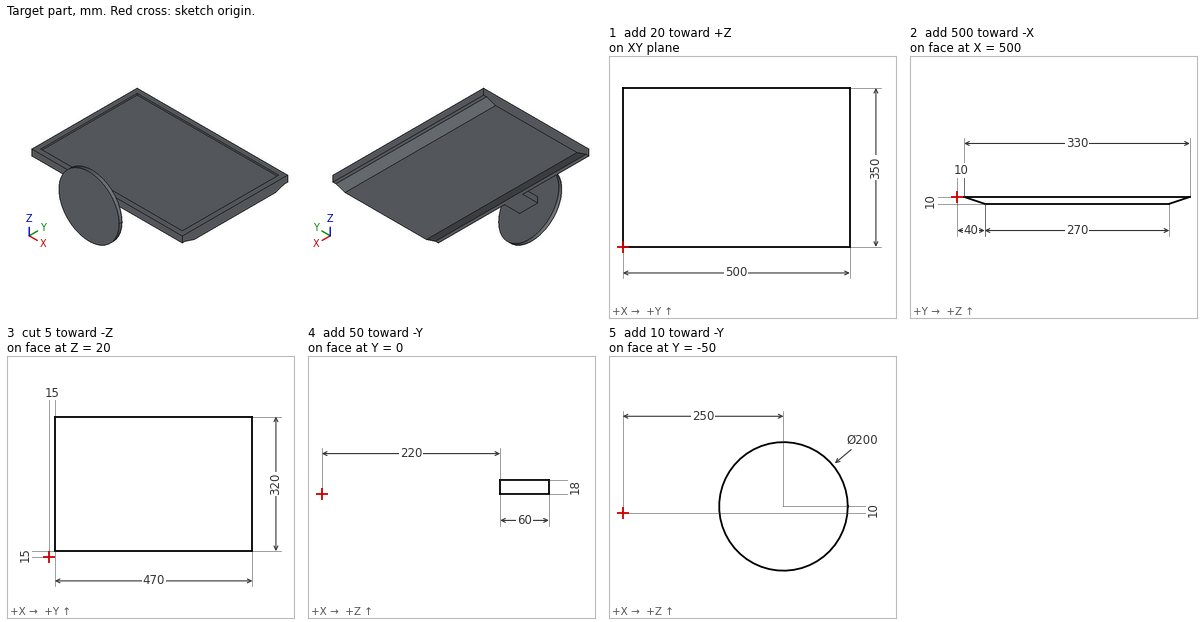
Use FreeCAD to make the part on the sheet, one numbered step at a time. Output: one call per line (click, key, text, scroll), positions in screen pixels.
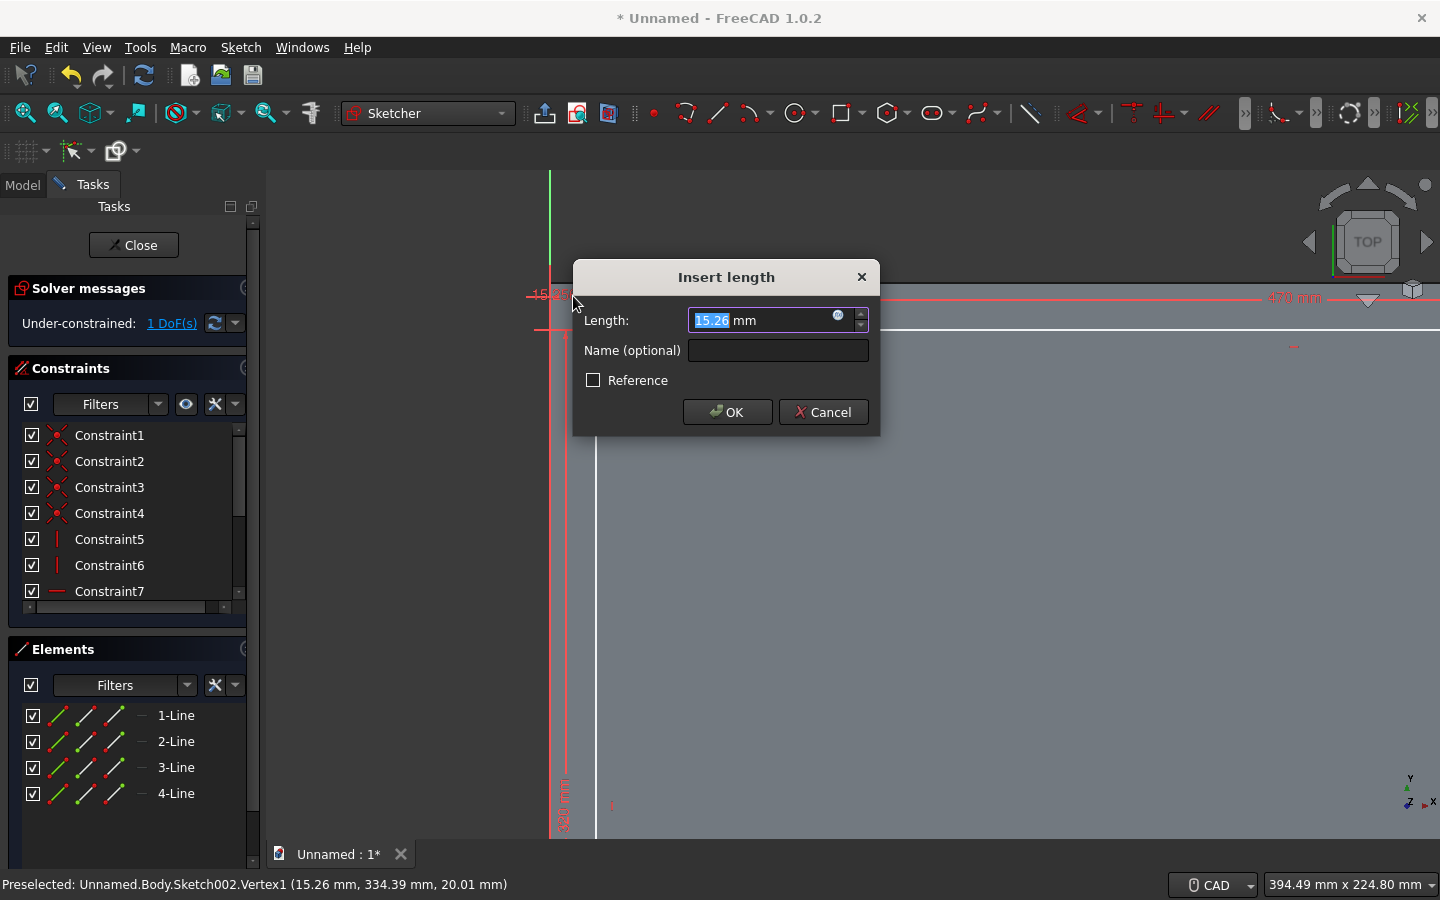
text(15)
key(Return)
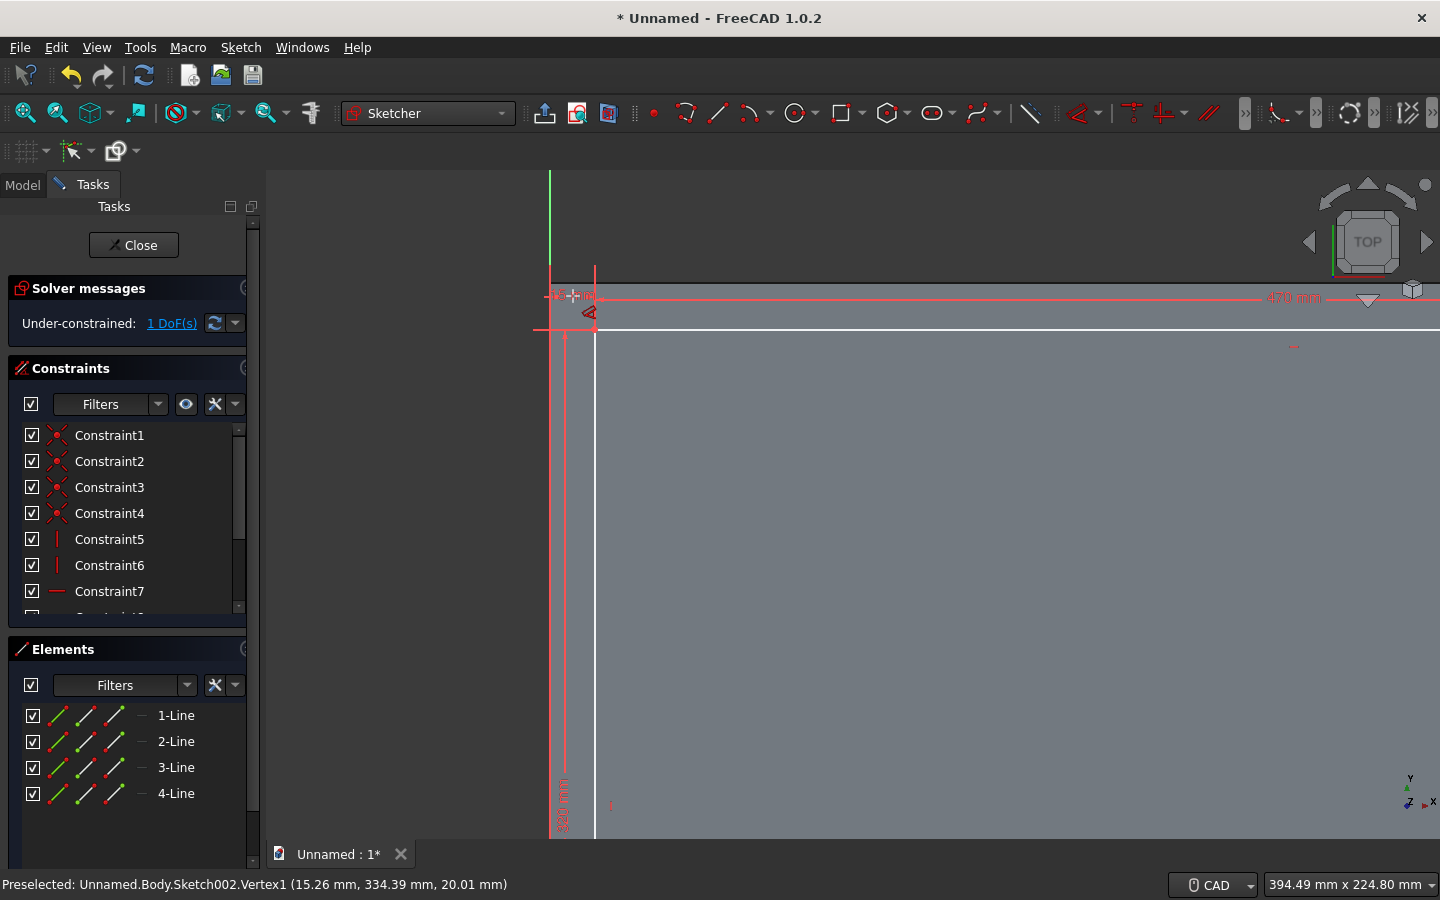
scroll(387, 242, down, 4)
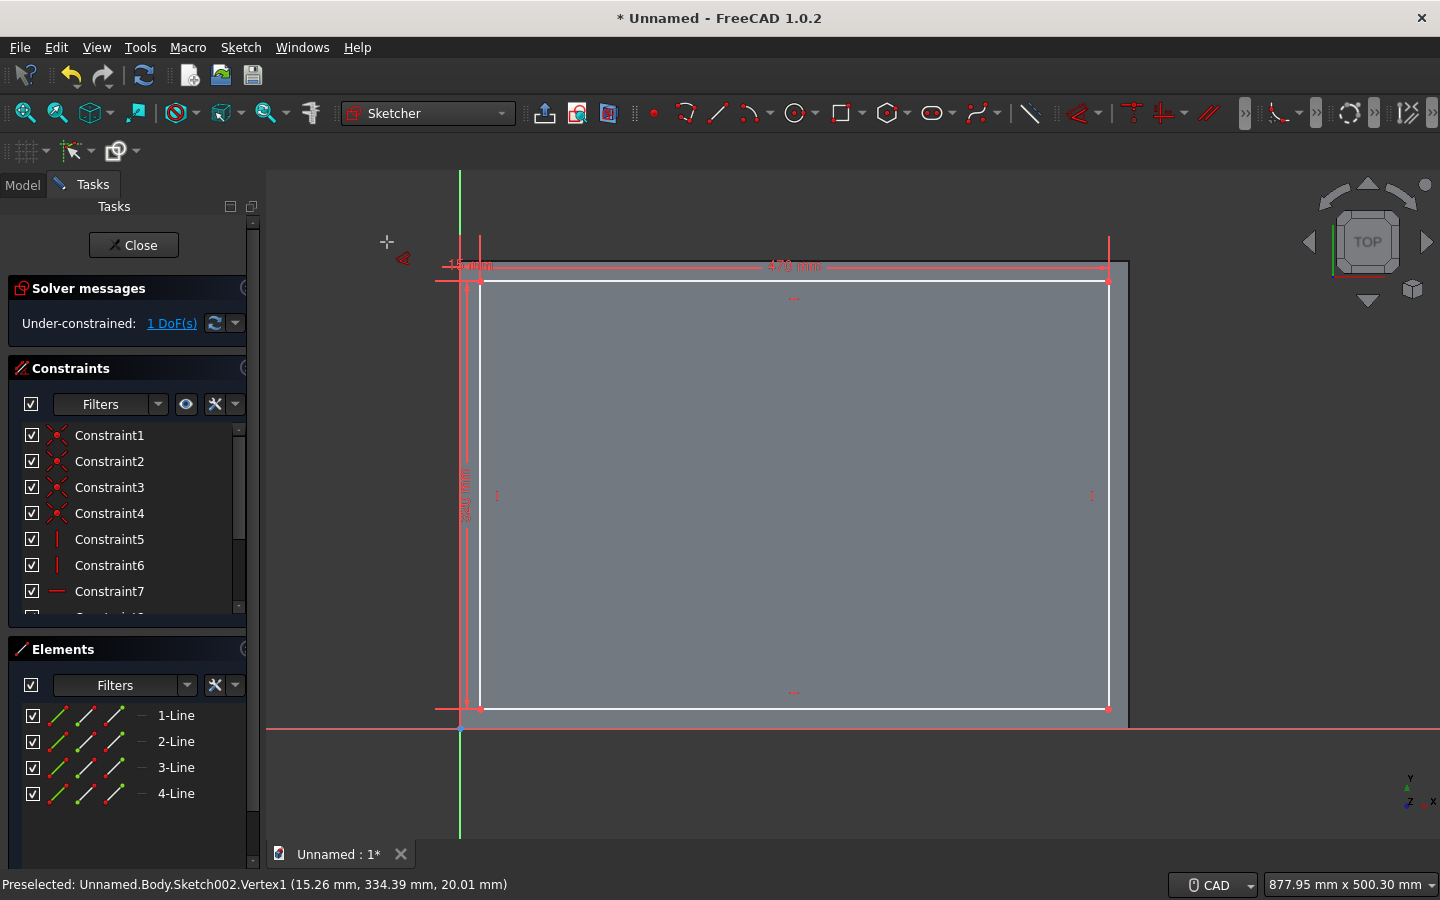
scroll(480, 709, up, 4)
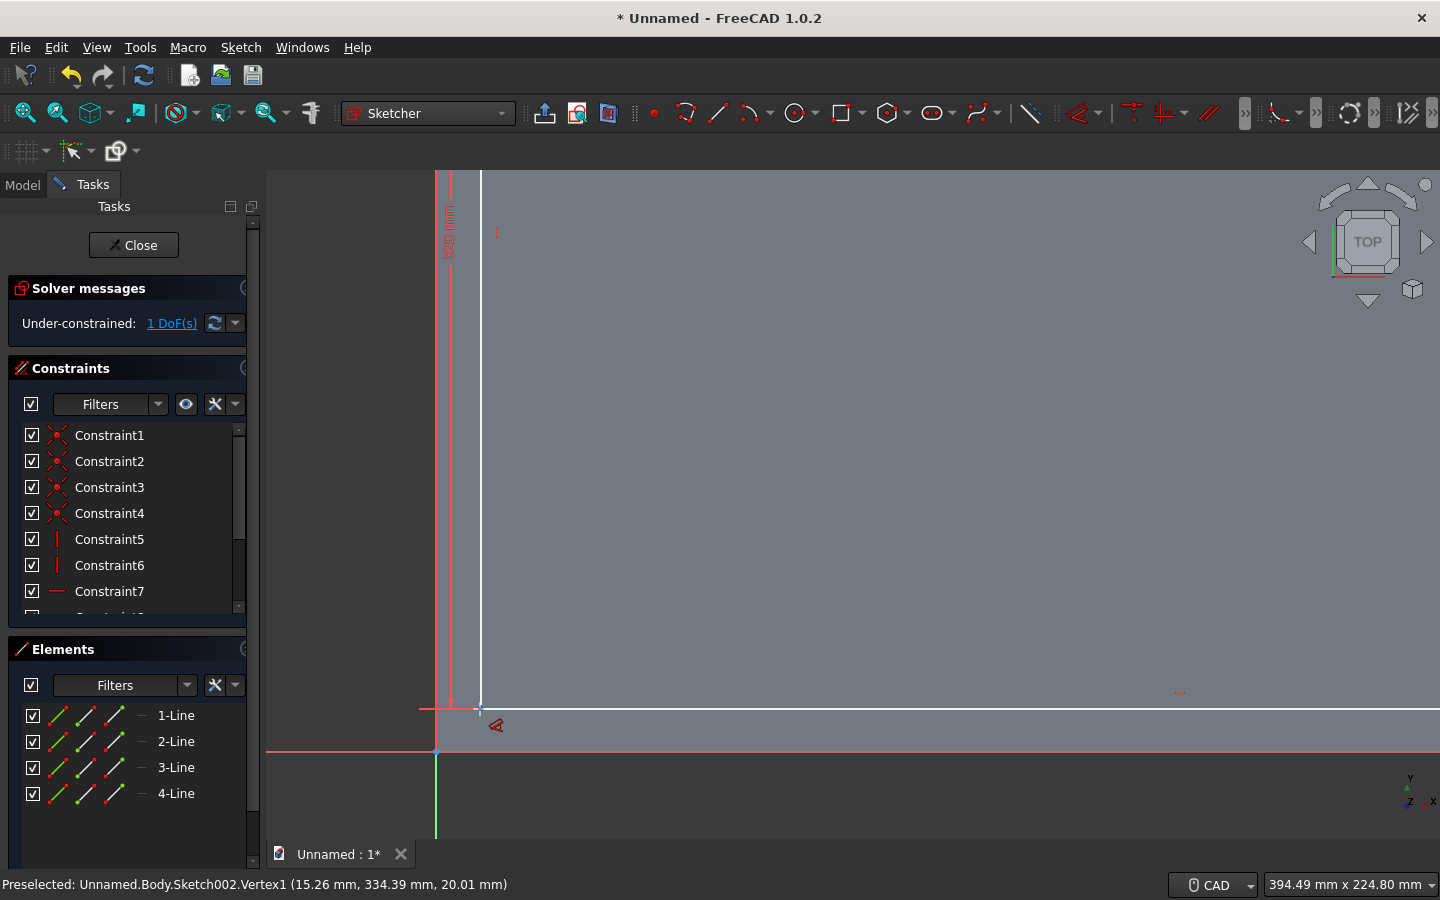
click(481, 709)
click(402, 730)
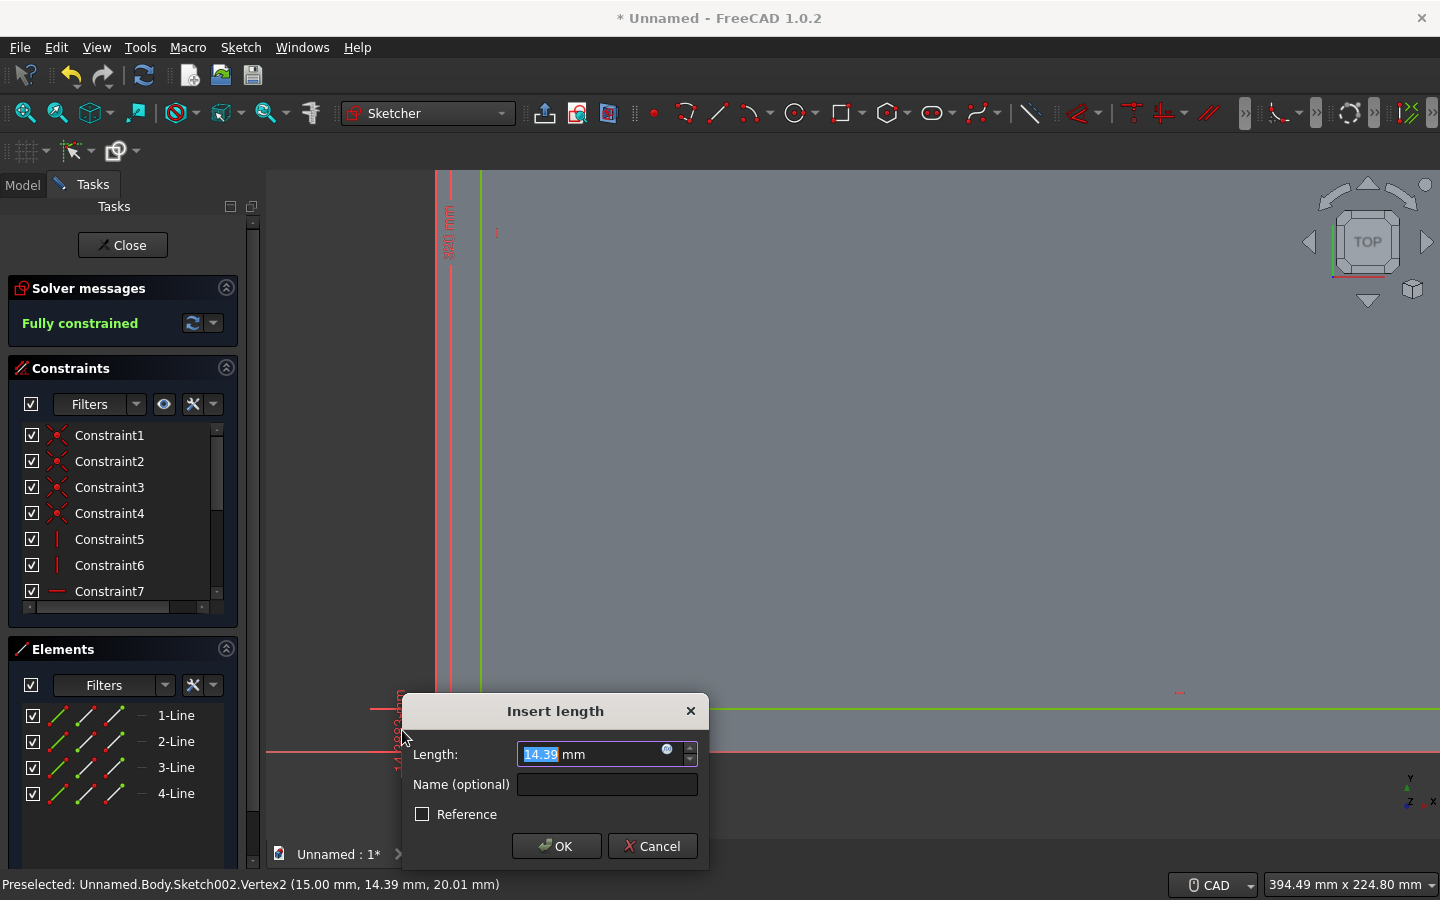
text(15)
key(Return)
key(Escape)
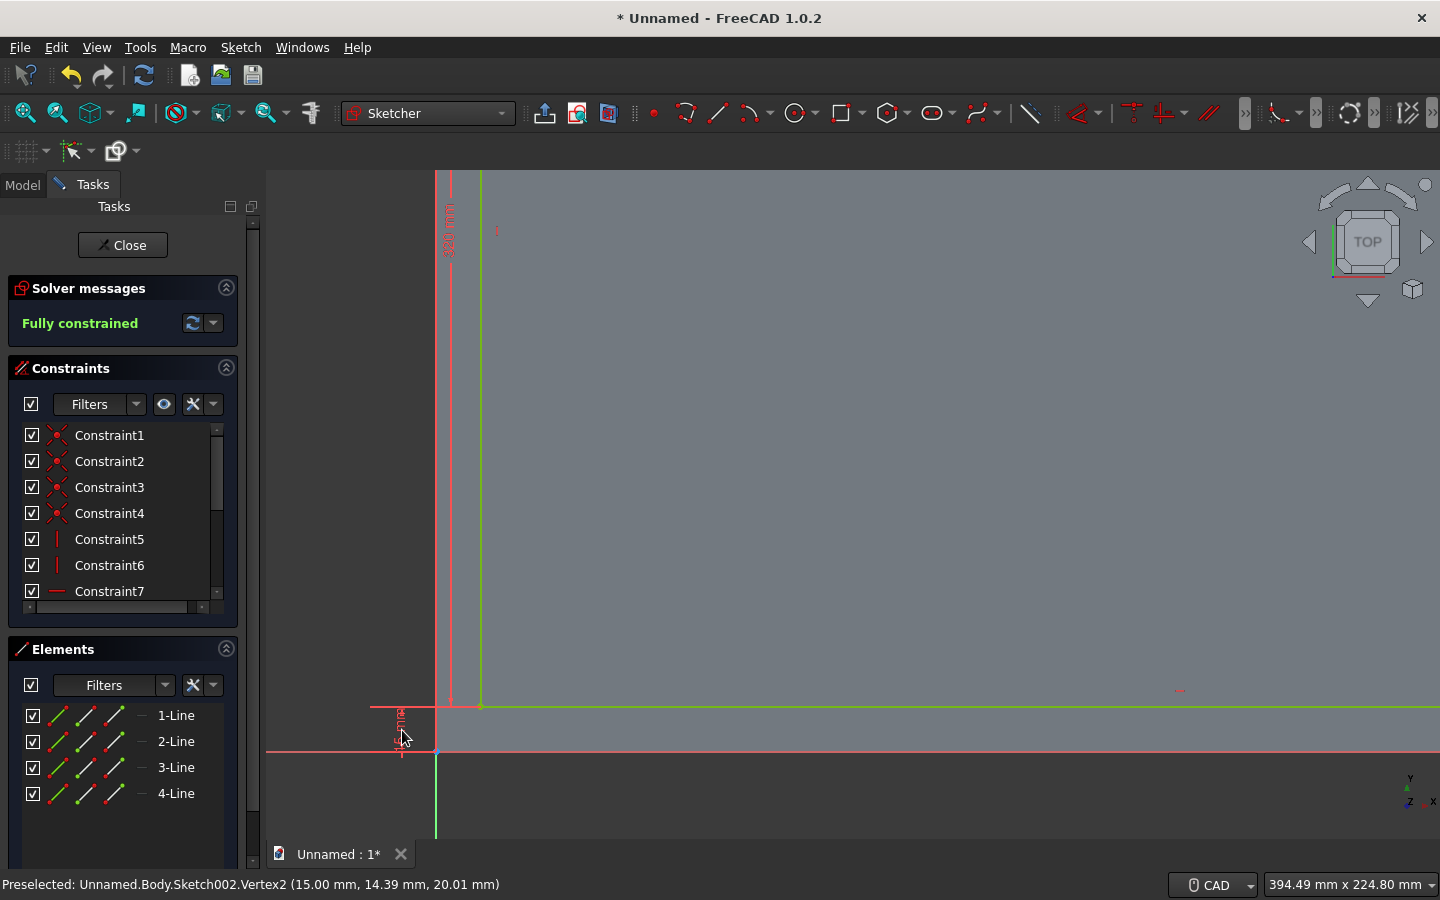
click(123, 245)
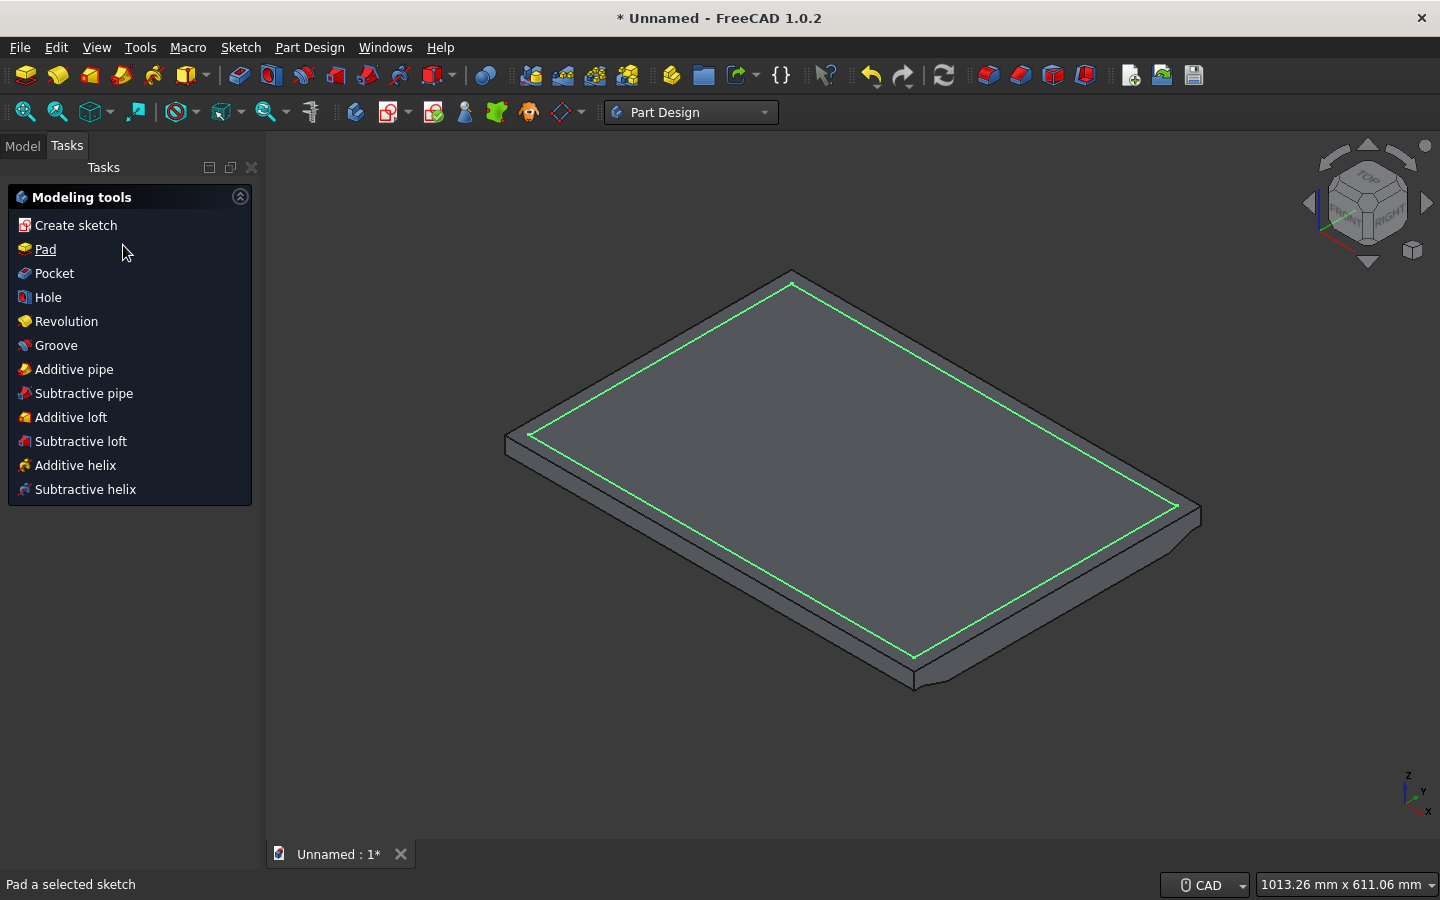
click(240, 76)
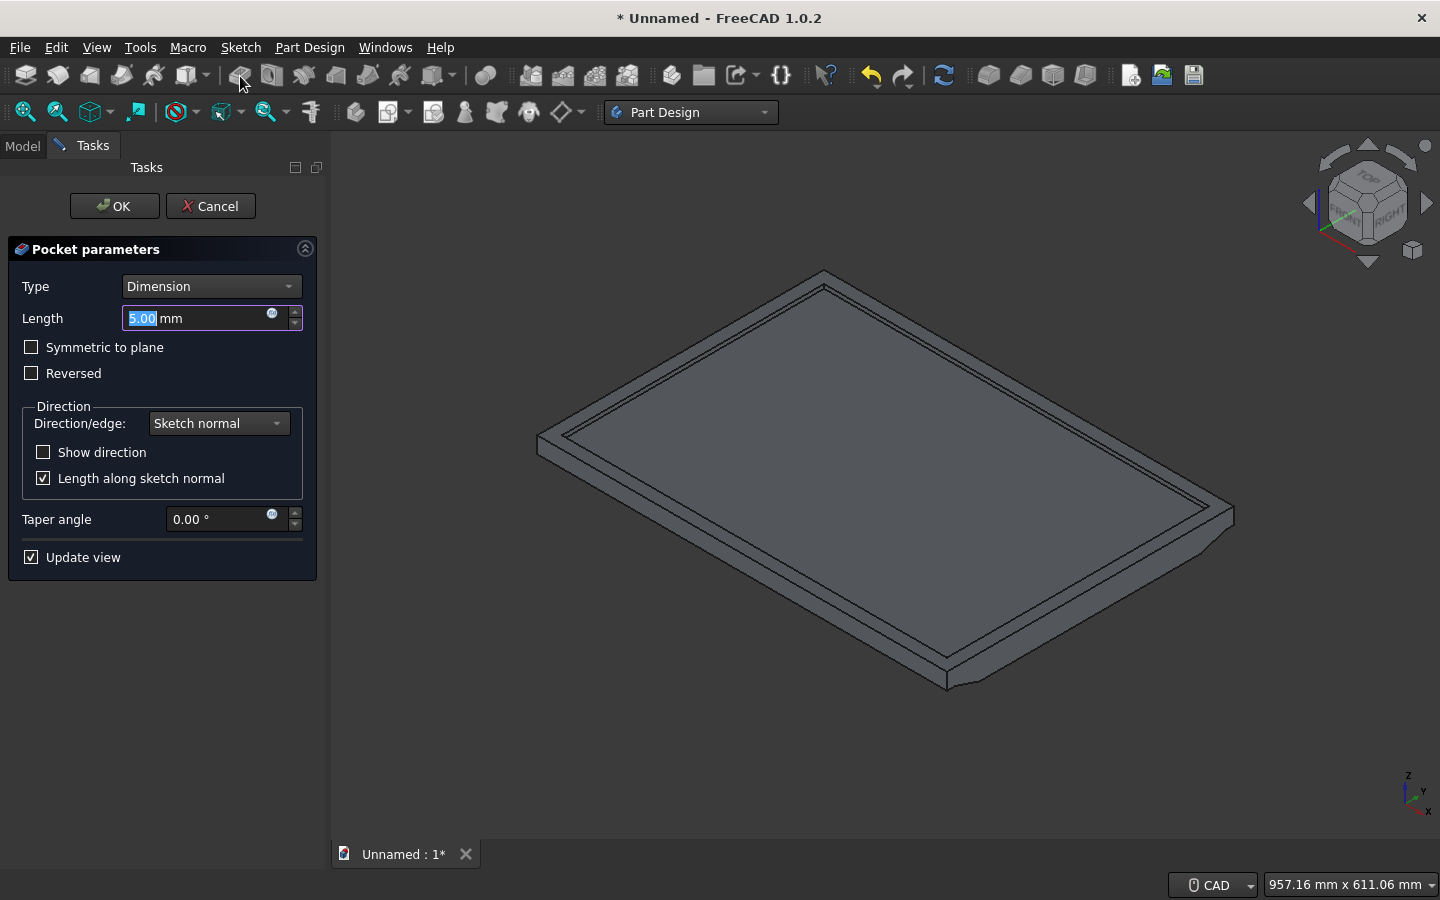
text(5)
key(Tab)